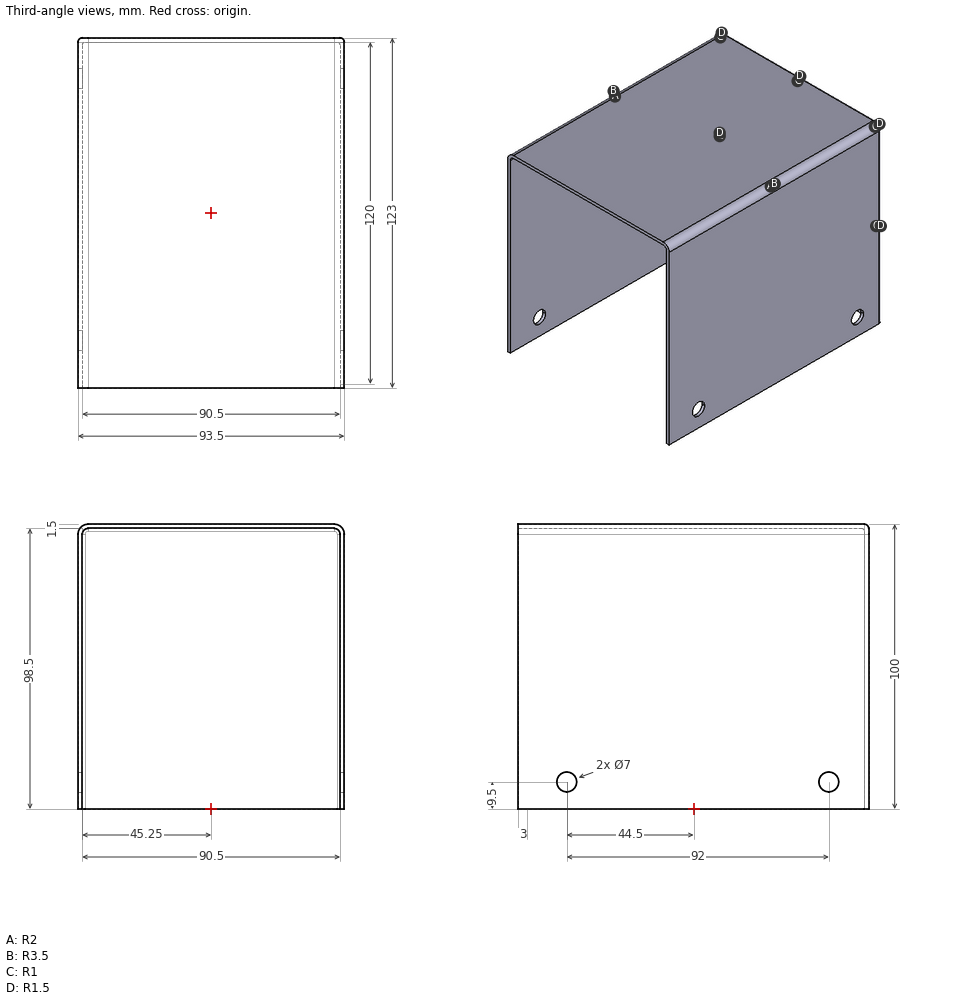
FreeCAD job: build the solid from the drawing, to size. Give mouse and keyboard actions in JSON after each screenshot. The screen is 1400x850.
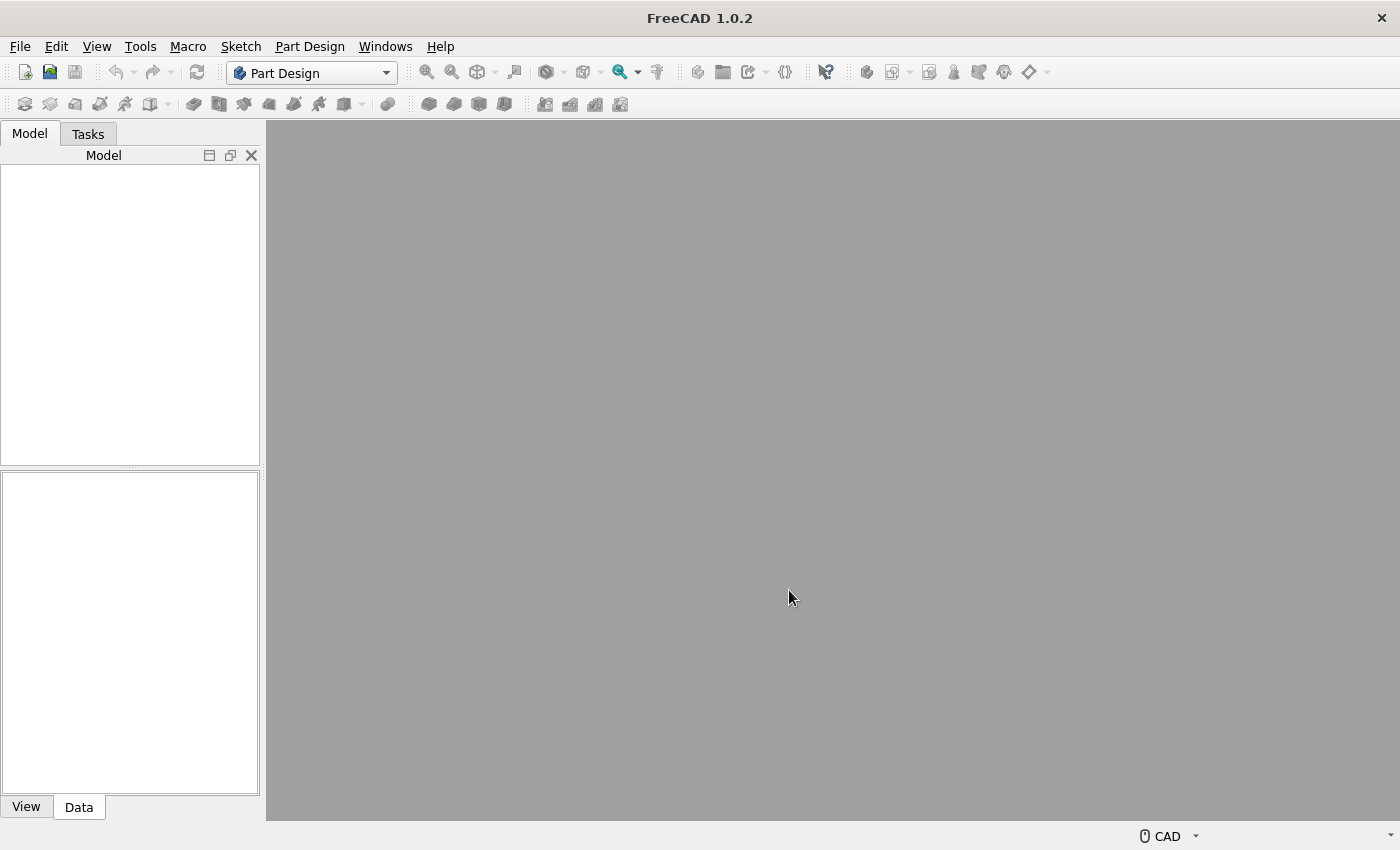
{"action": "left_click", "coordinate": [25, 72]}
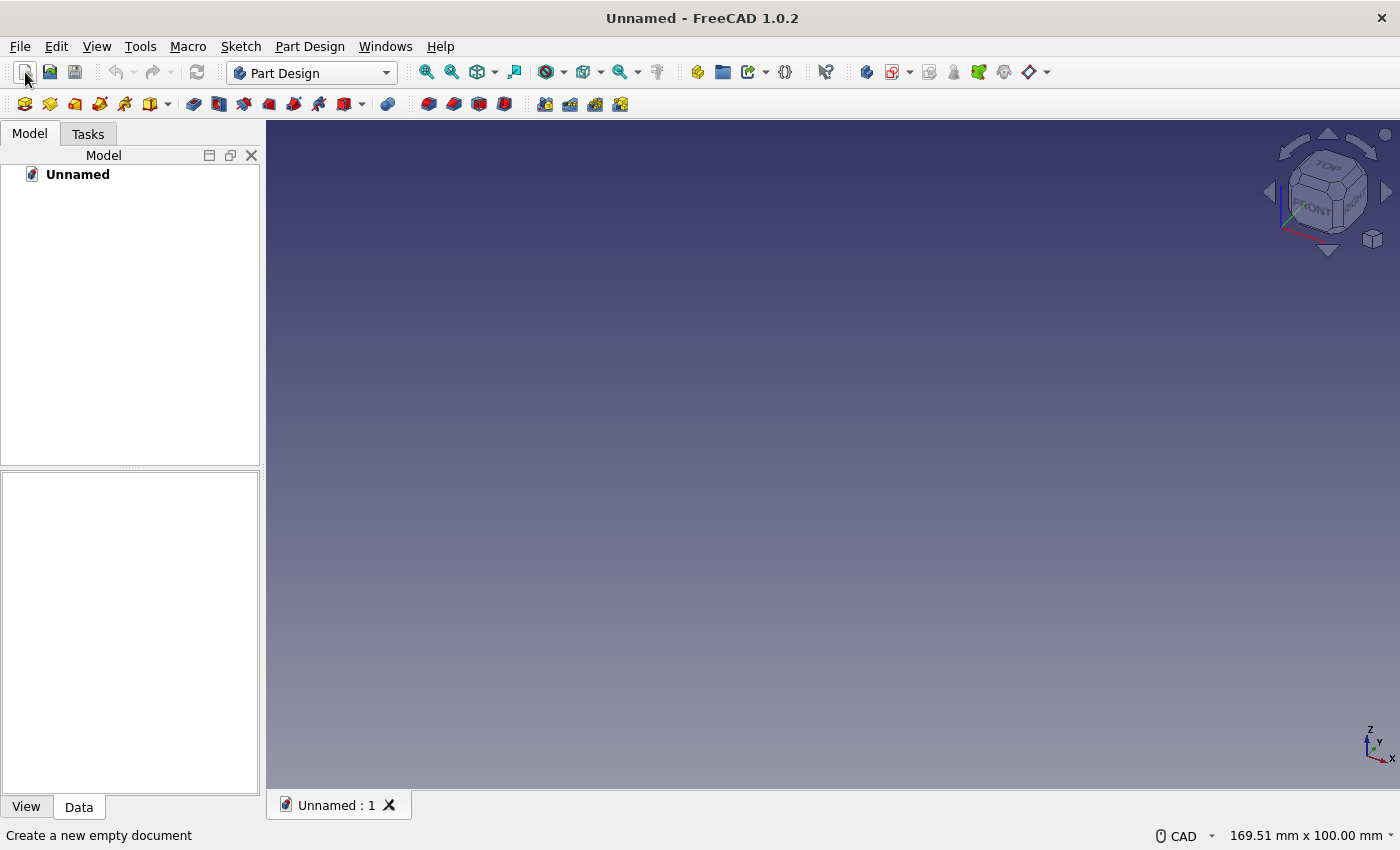
{"action": "left_click", "coordinate": [892, 72]}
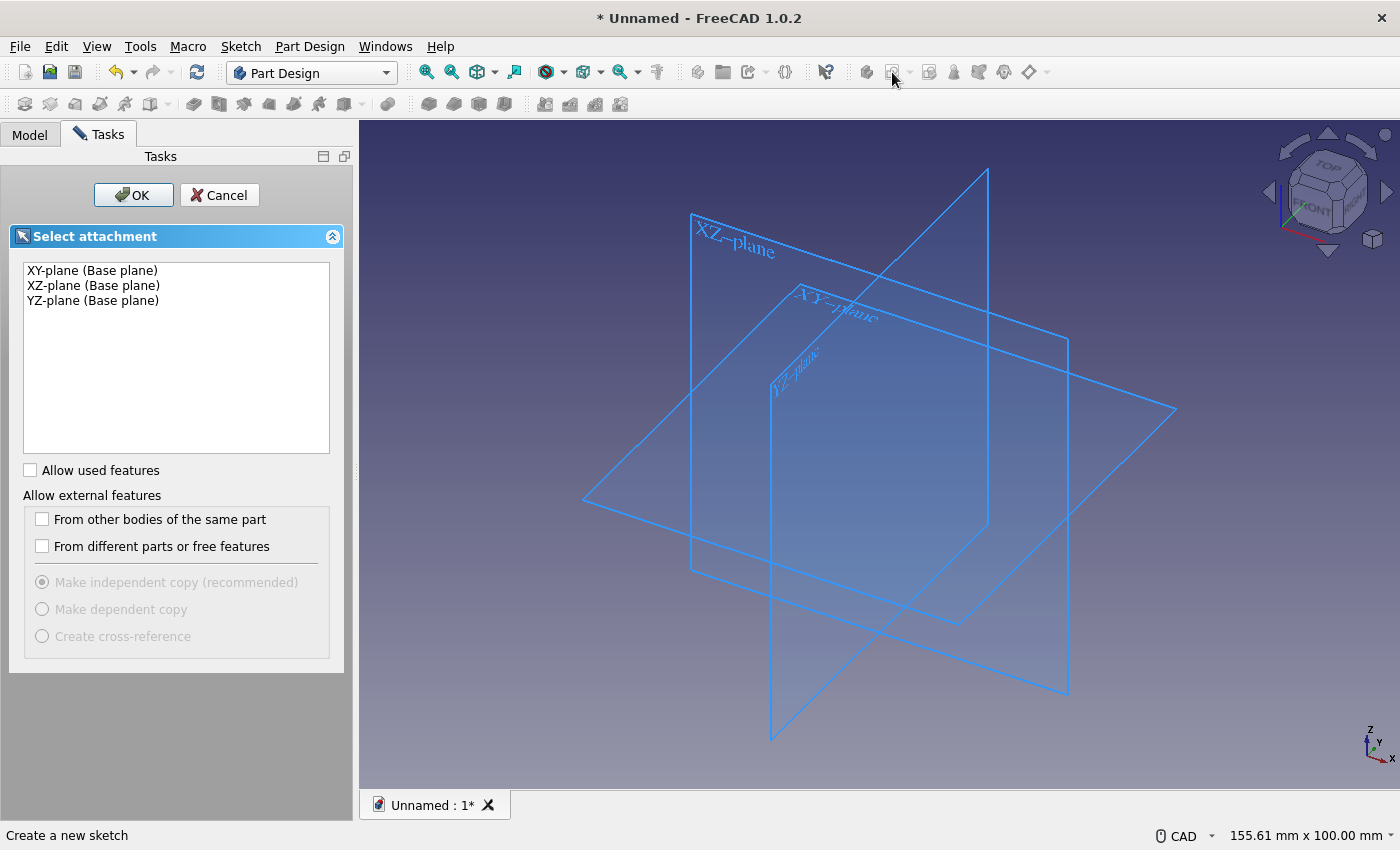
{"action": "left_click", "coordinate": [84, 270]}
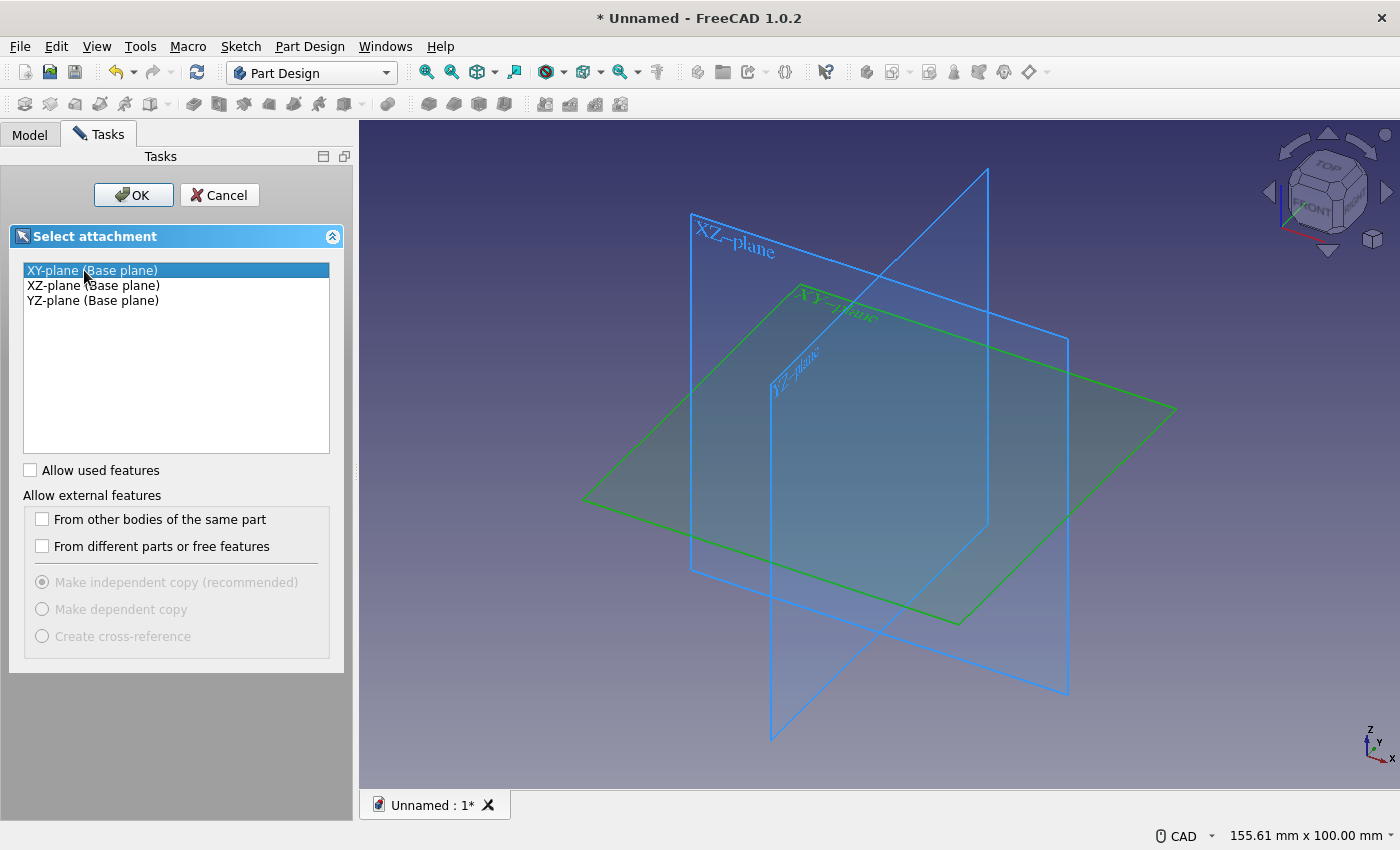
{"action": "left_click", "coordinate": [134, 195]}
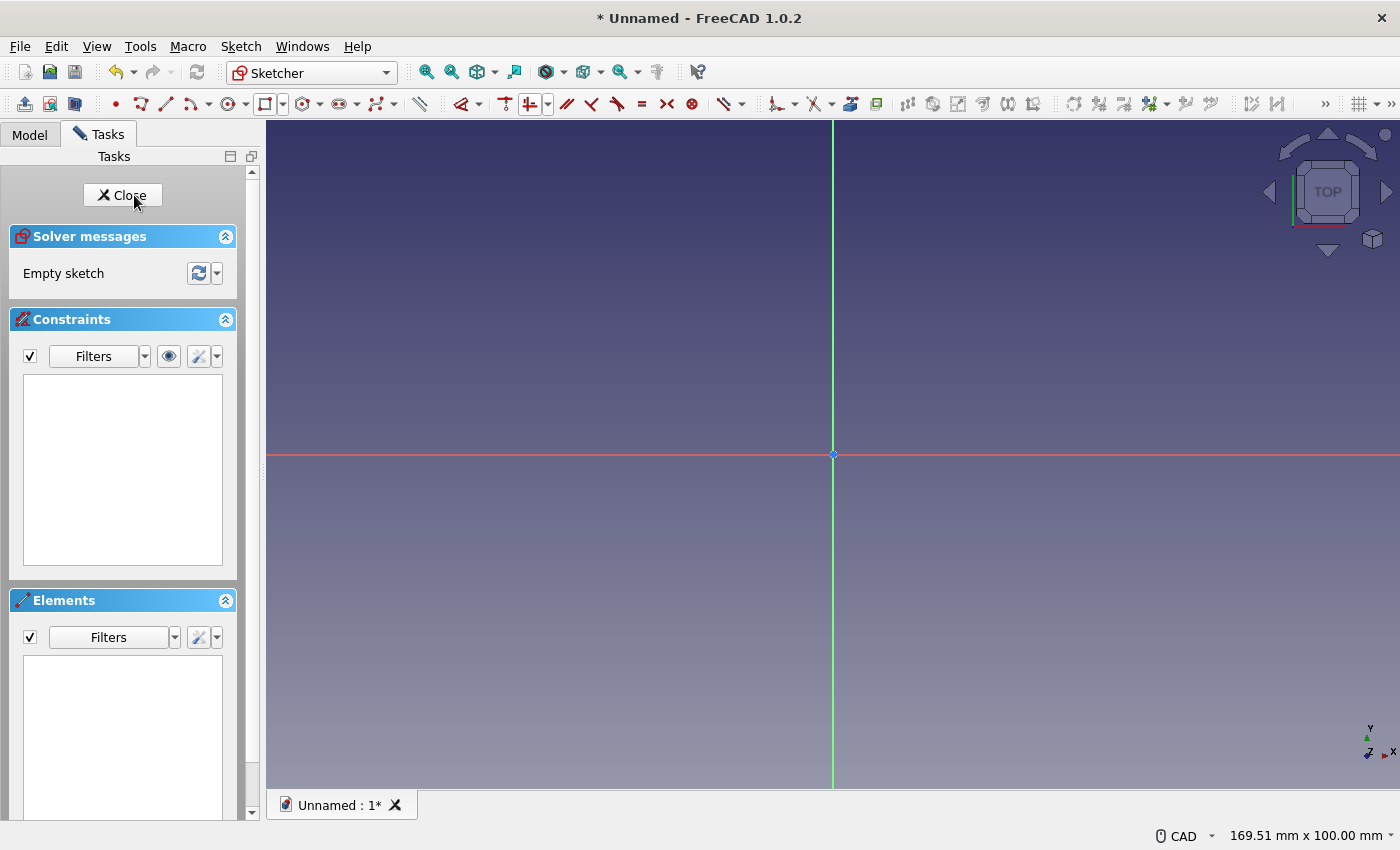
{"action": "scroll", "coordinate": [681, 454], "scroll_direction": "down", "scroll_amount": 3}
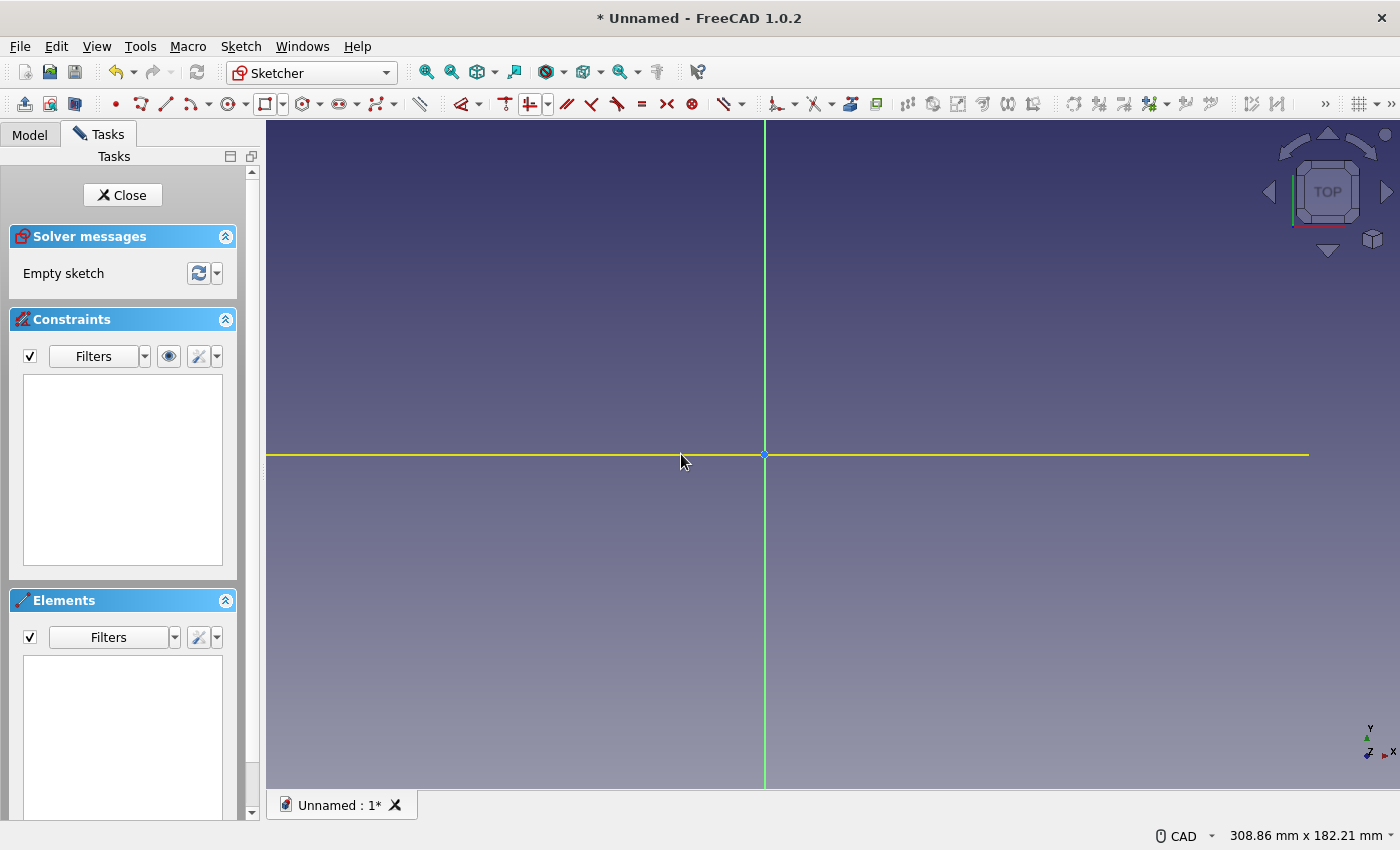
{"action": "left_click", "coordinate": [282, 104]}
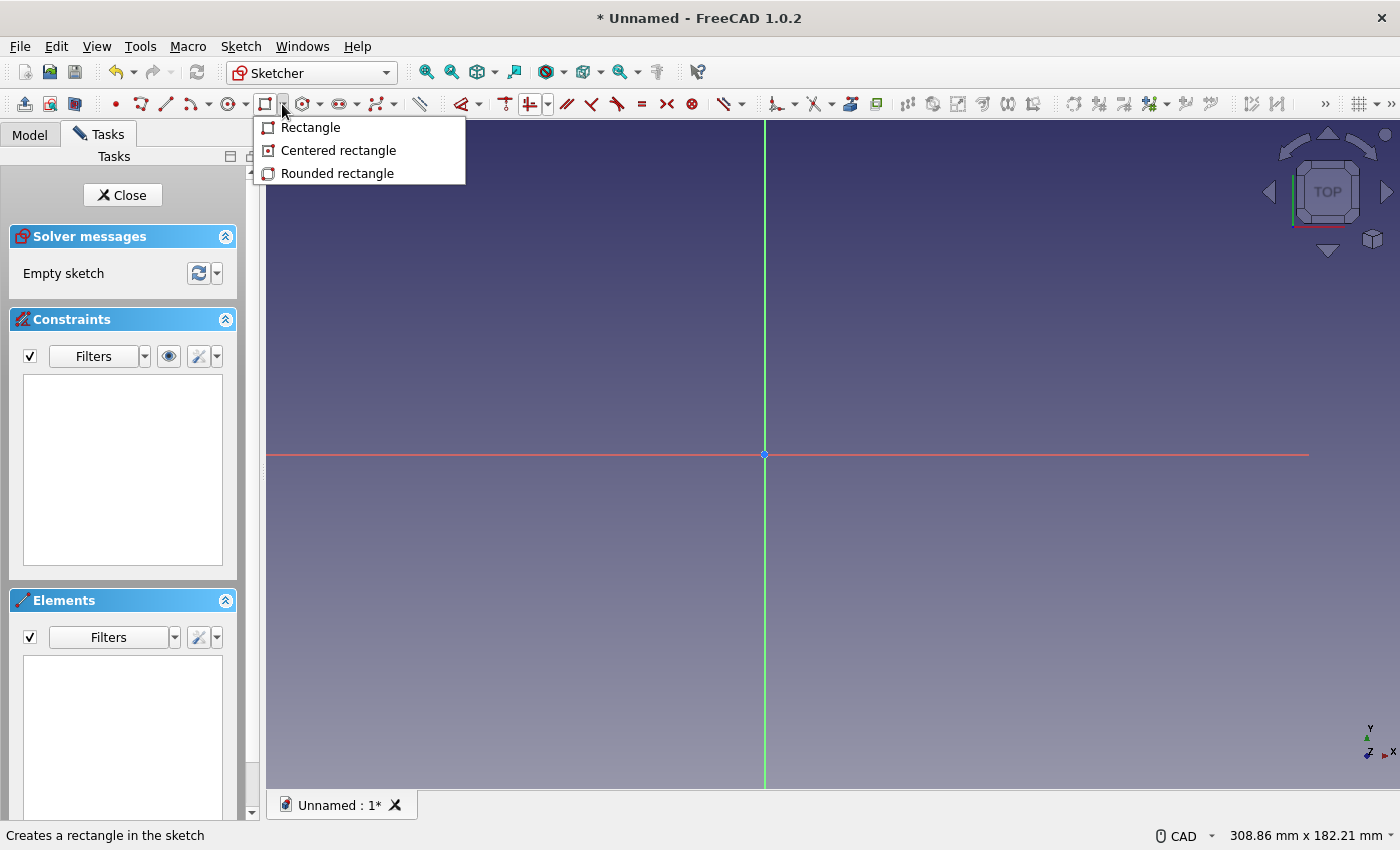
{"action": "left_click", "coordinate": [360, 150]}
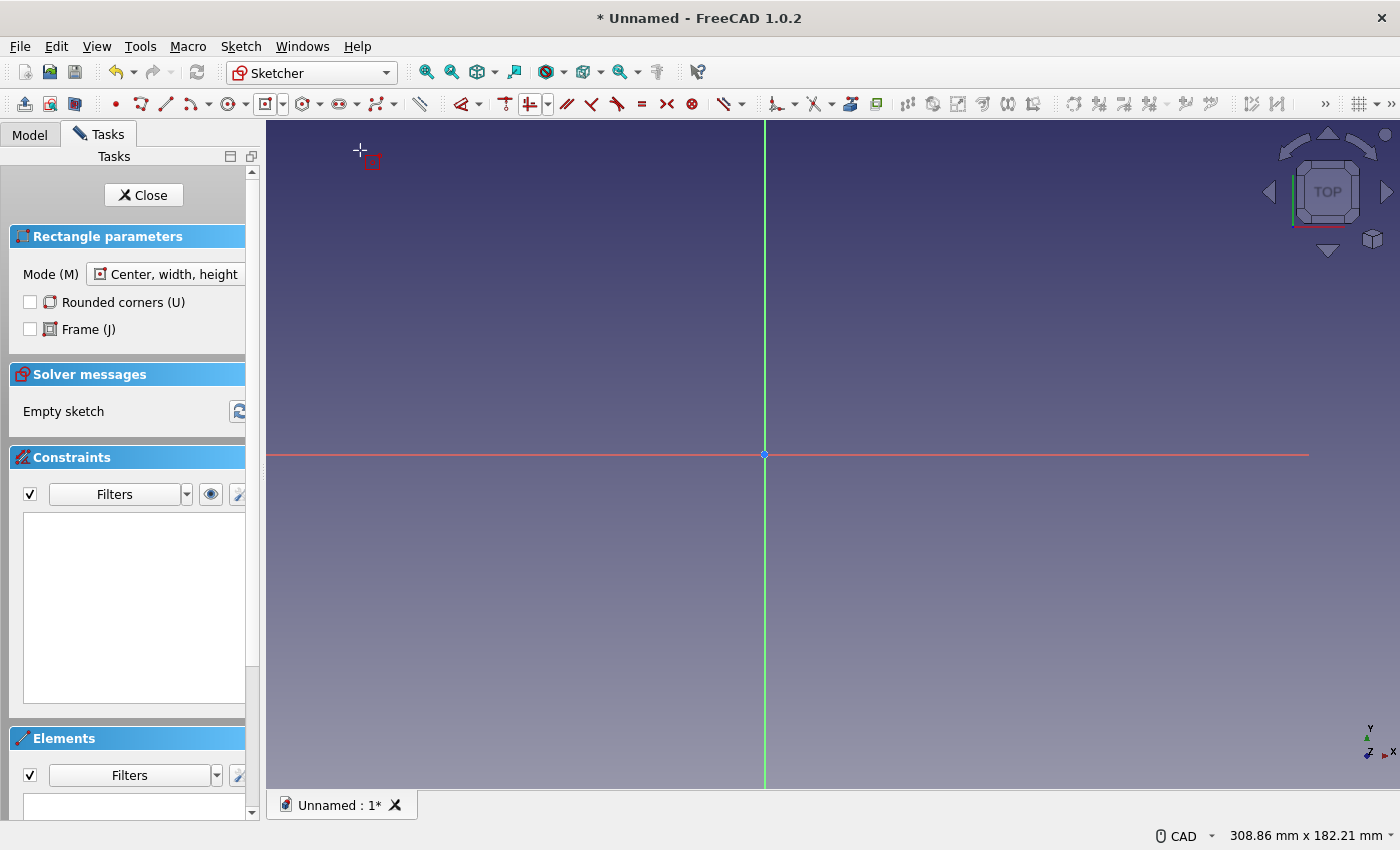
{"action": "left_click", "coordinate": [765, 454]}
{"action": "mouse_move", "coordinate": [936, 229]}